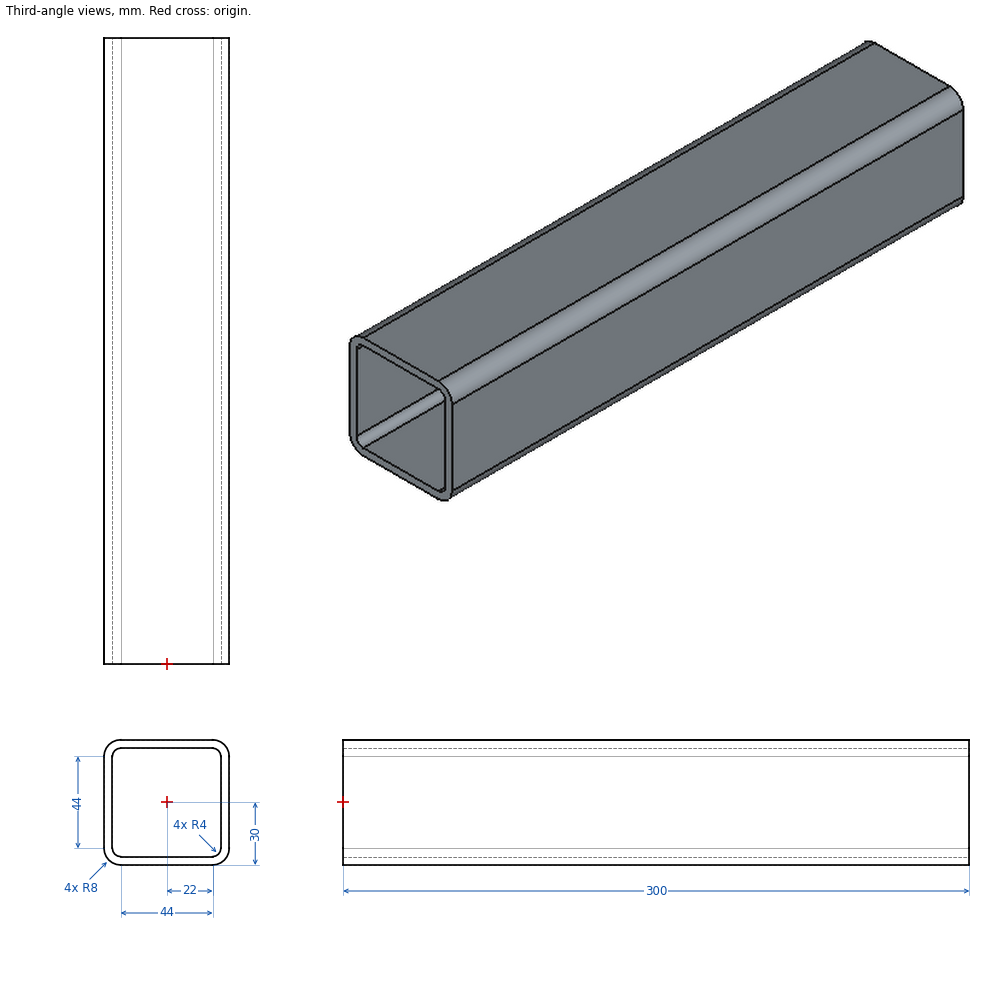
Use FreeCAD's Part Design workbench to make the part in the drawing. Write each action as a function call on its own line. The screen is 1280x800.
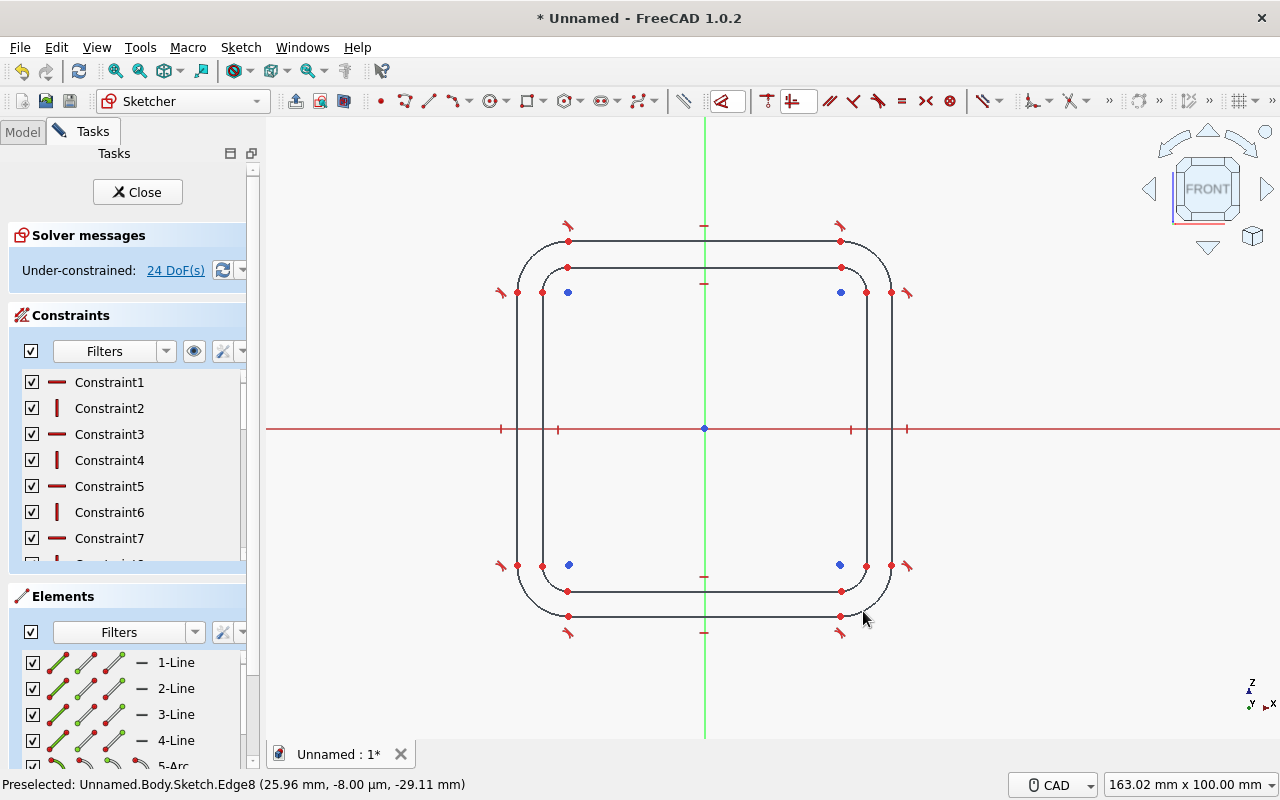
click(650, 592)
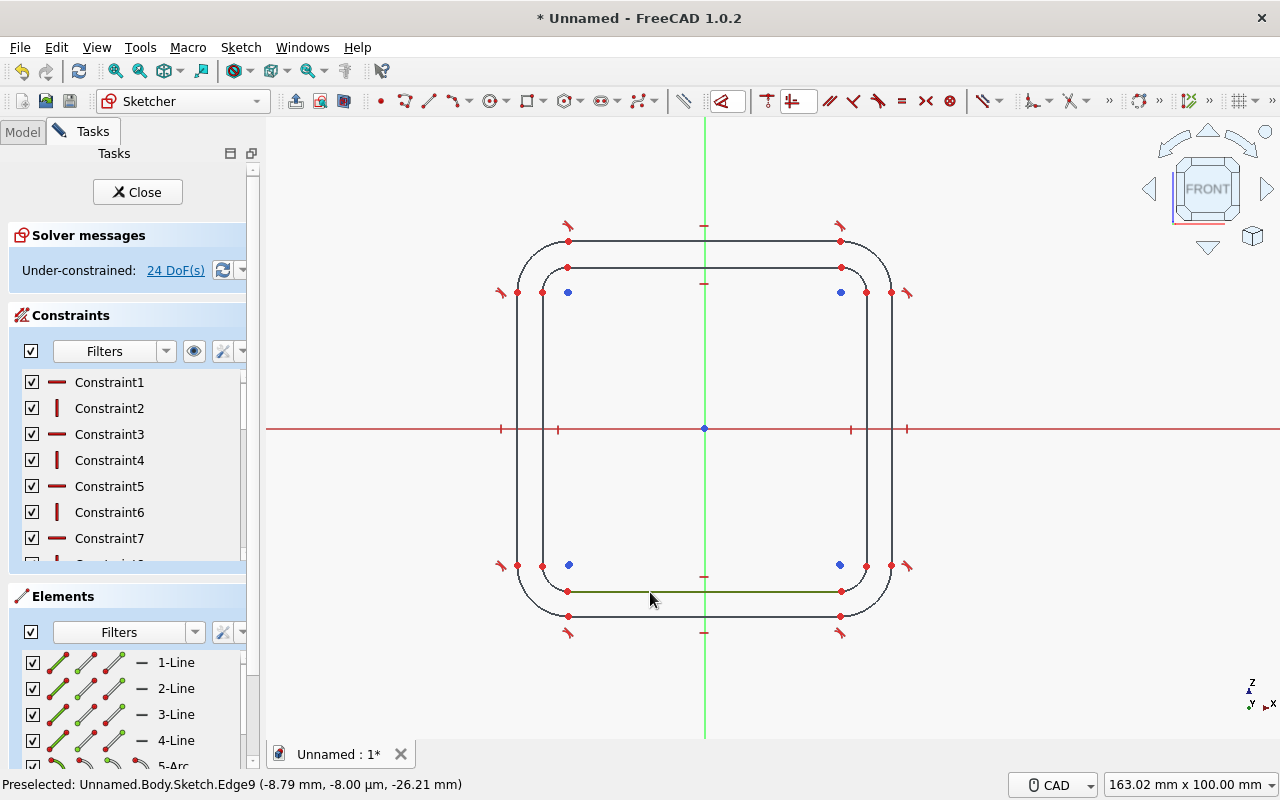
click(853, 588)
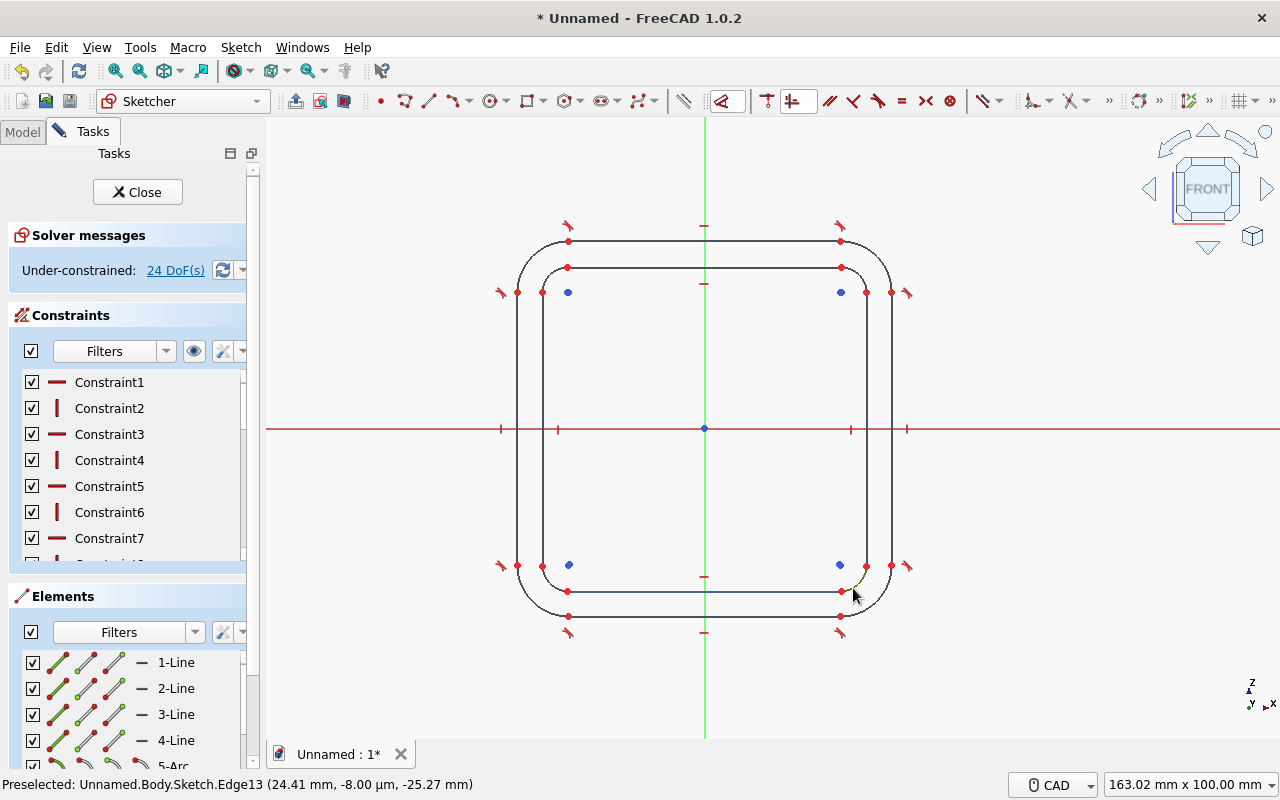
click(878, 102)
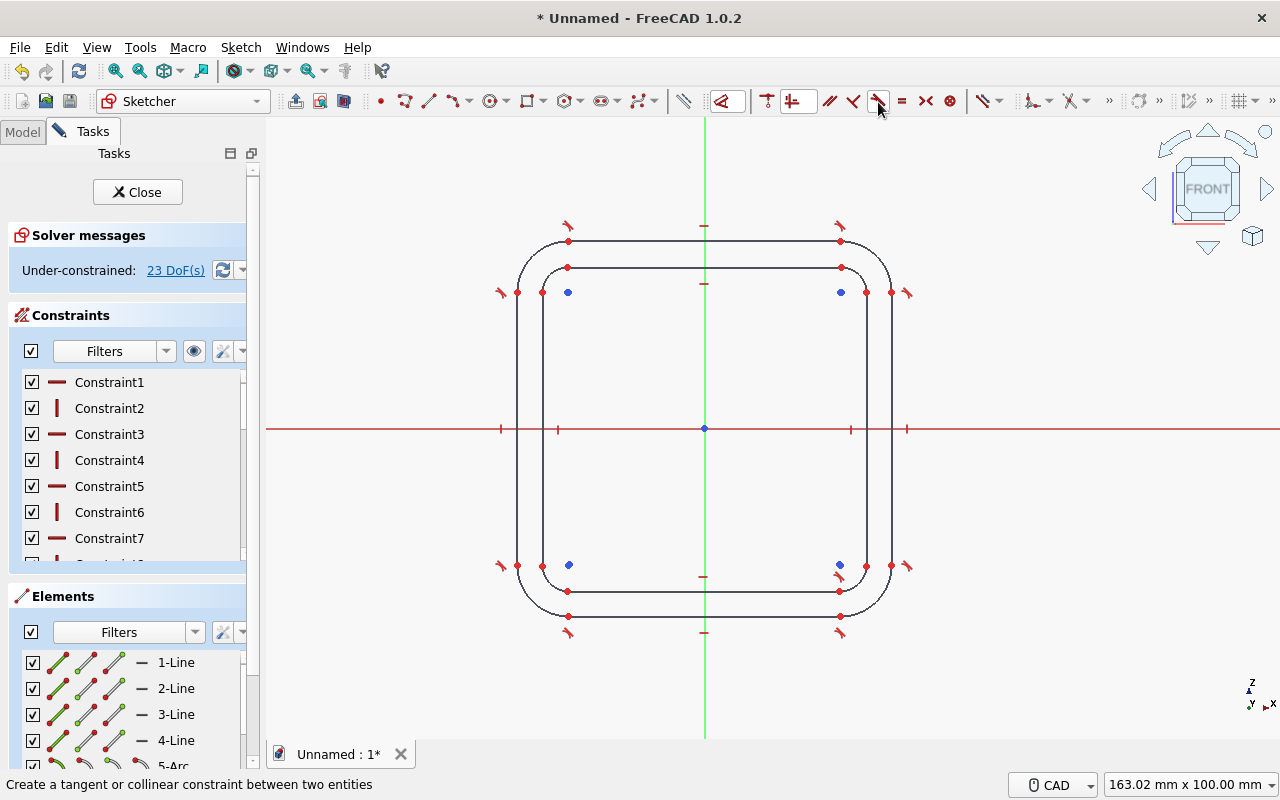
click(649, 592)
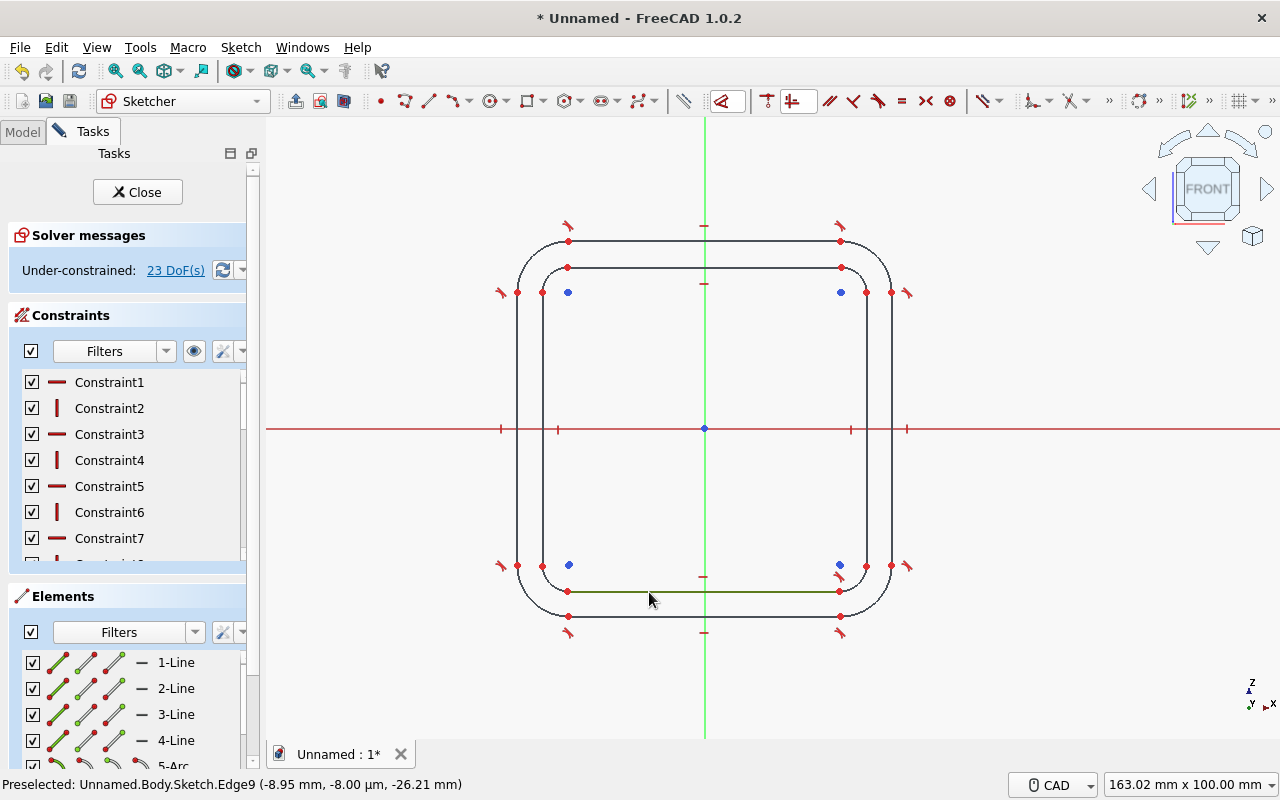
click(546, 578)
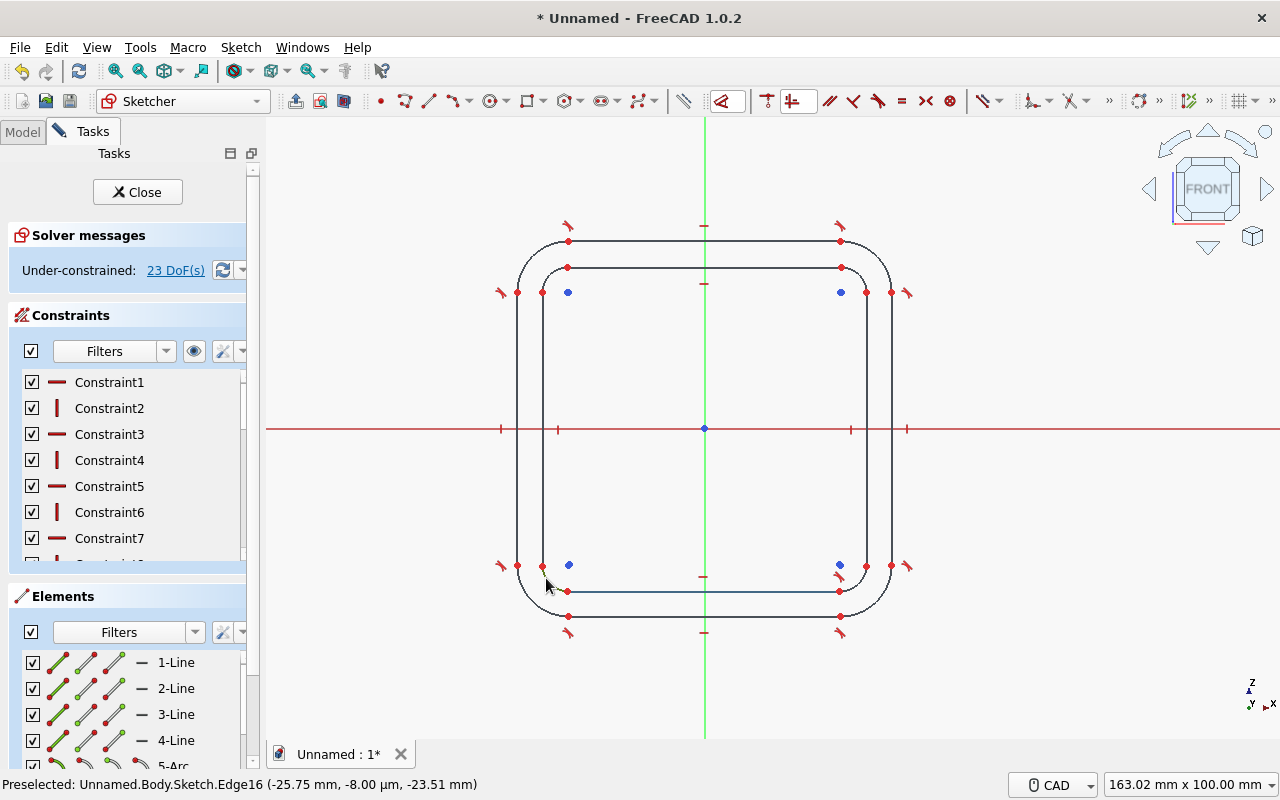
click(878, 102)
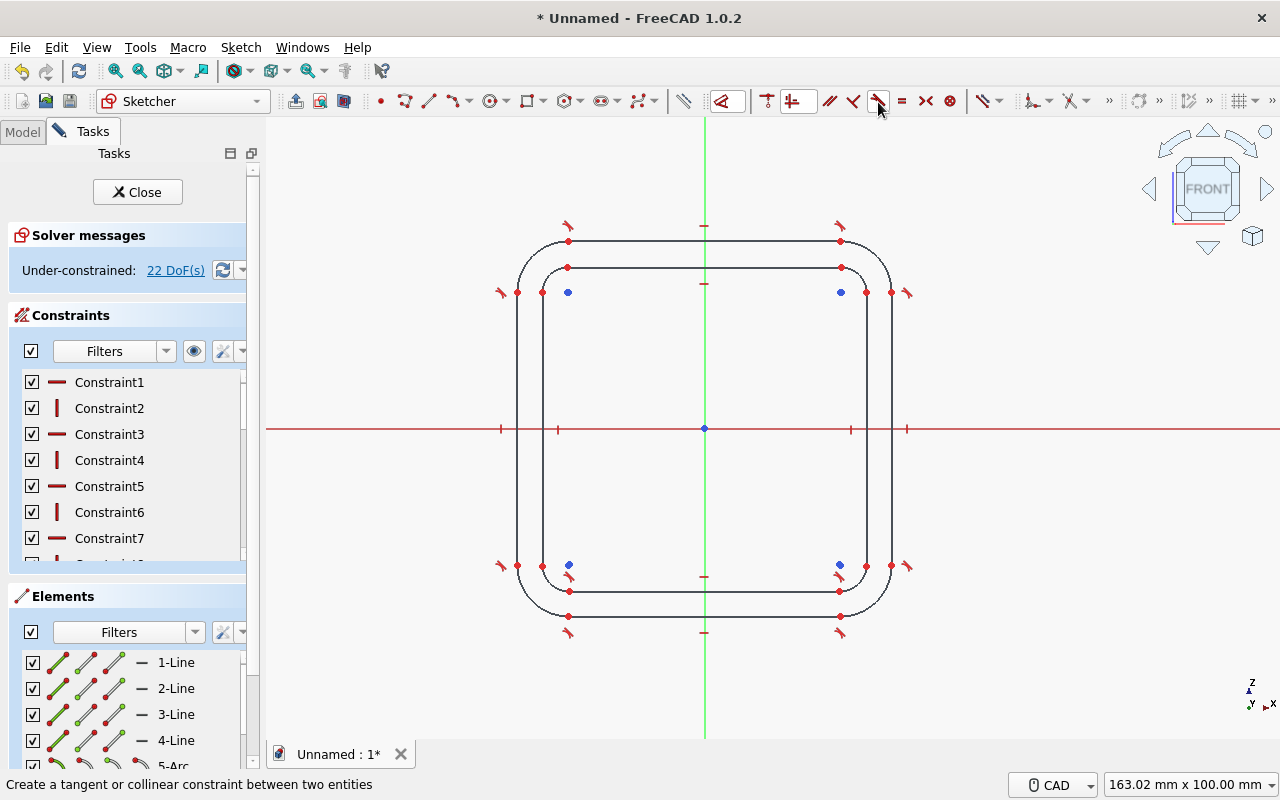
click(867, 484)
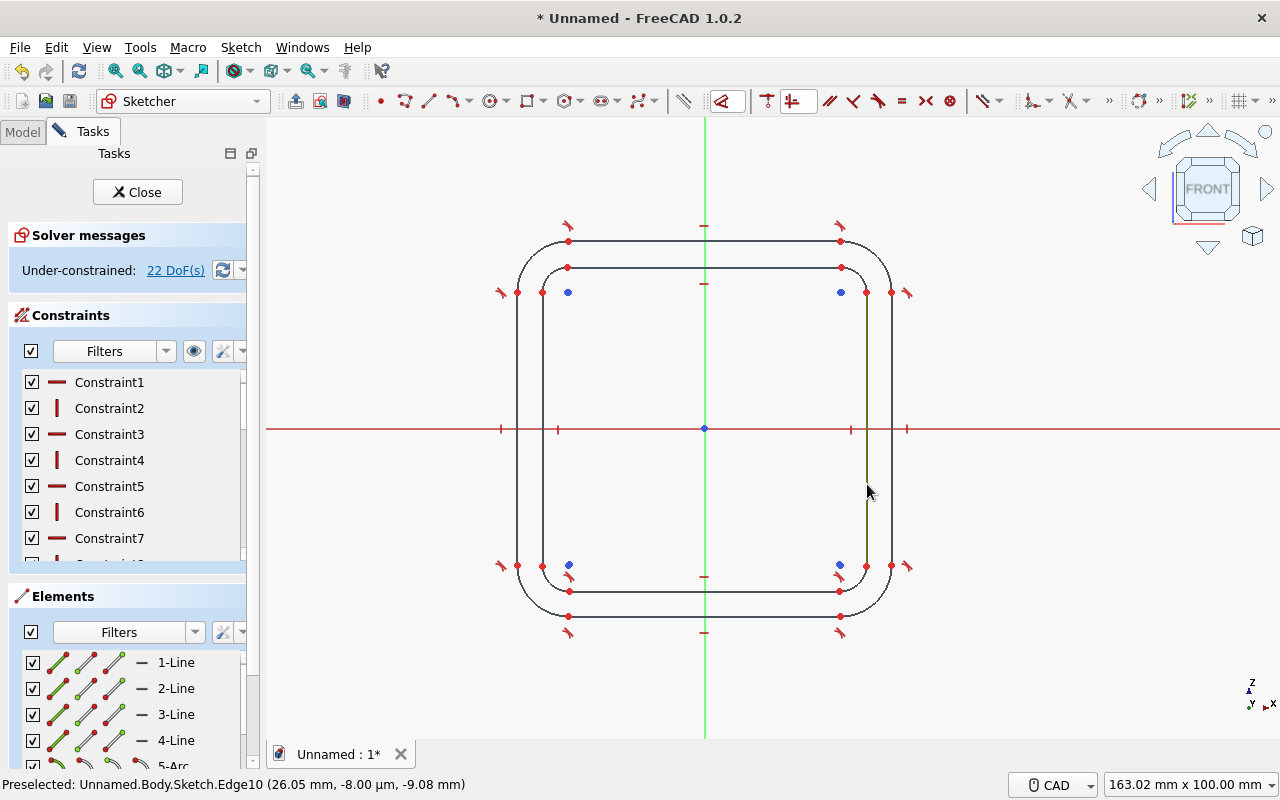
click(851, 589)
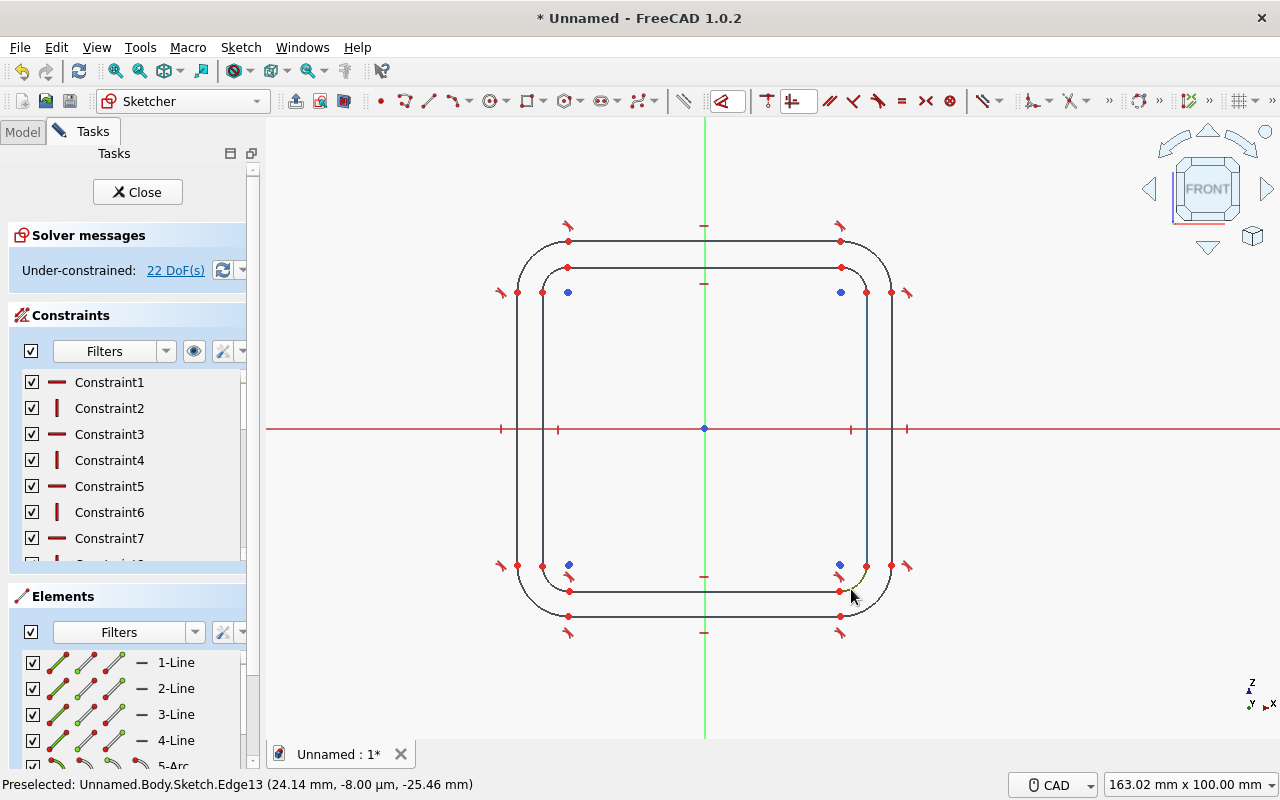
key(t)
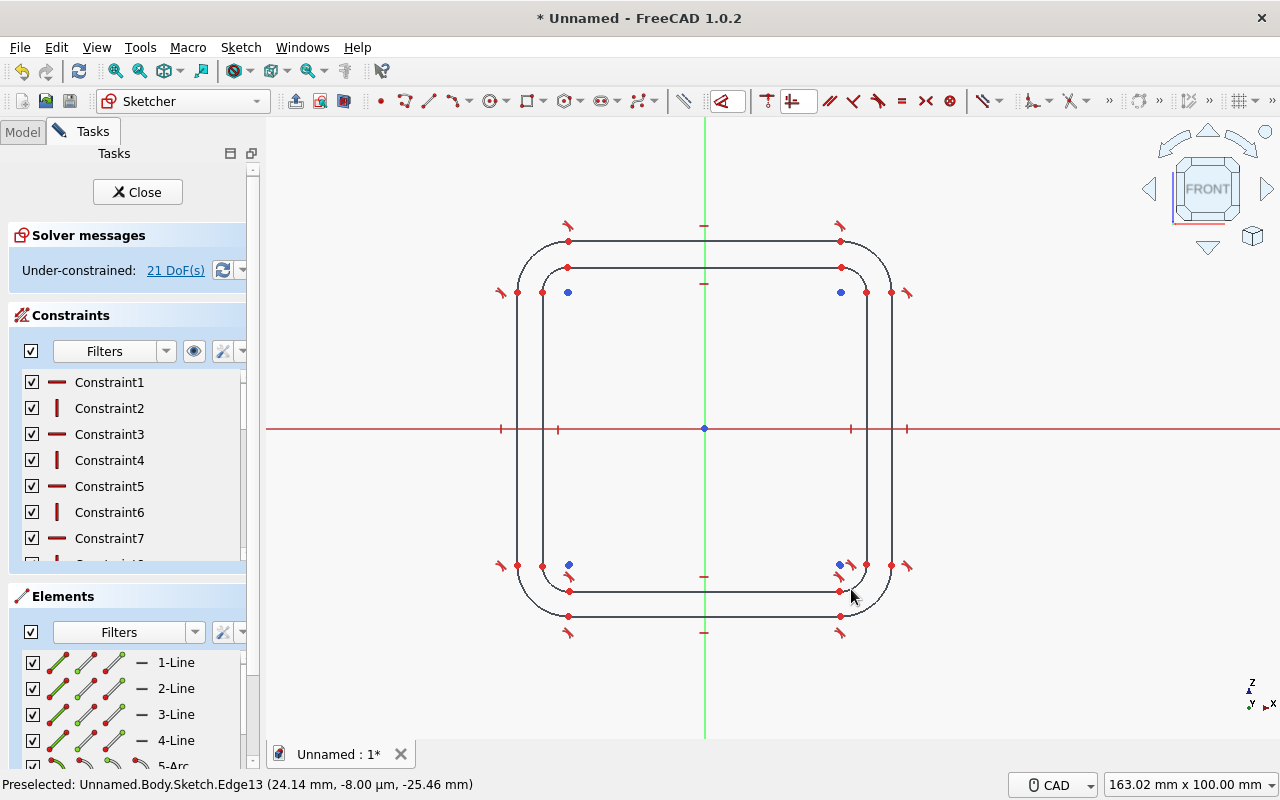
click(867, 483)